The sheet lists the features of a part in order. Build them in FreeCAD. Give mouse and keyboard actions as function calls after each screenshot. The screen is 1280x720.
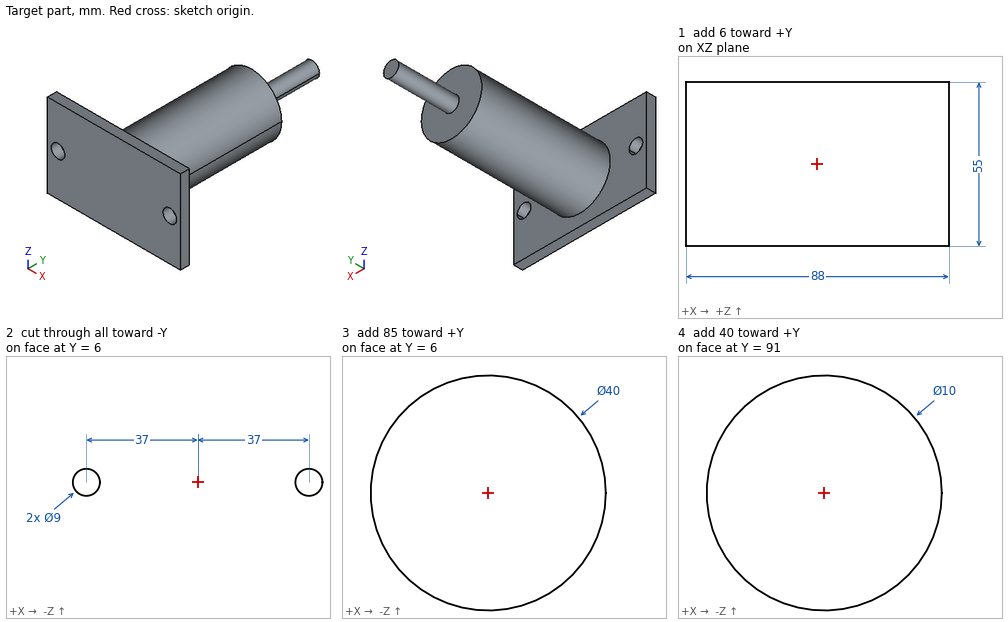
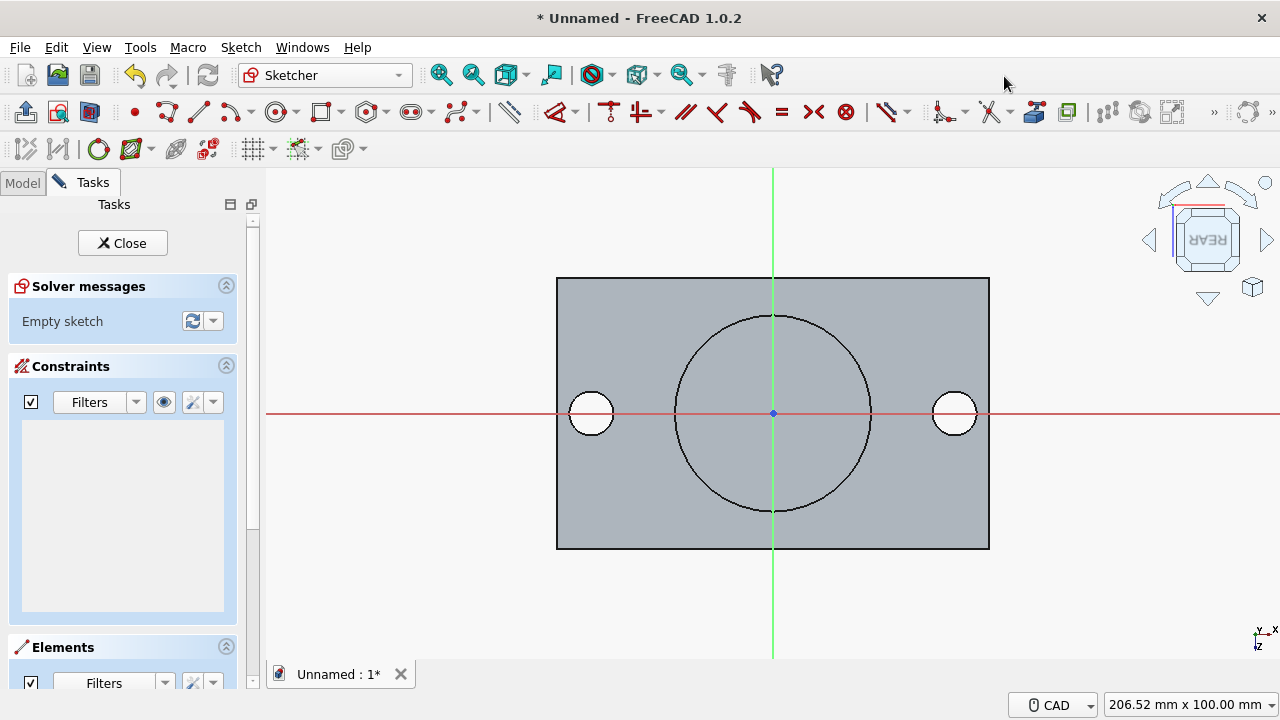
scroll(787, 413, up, 9)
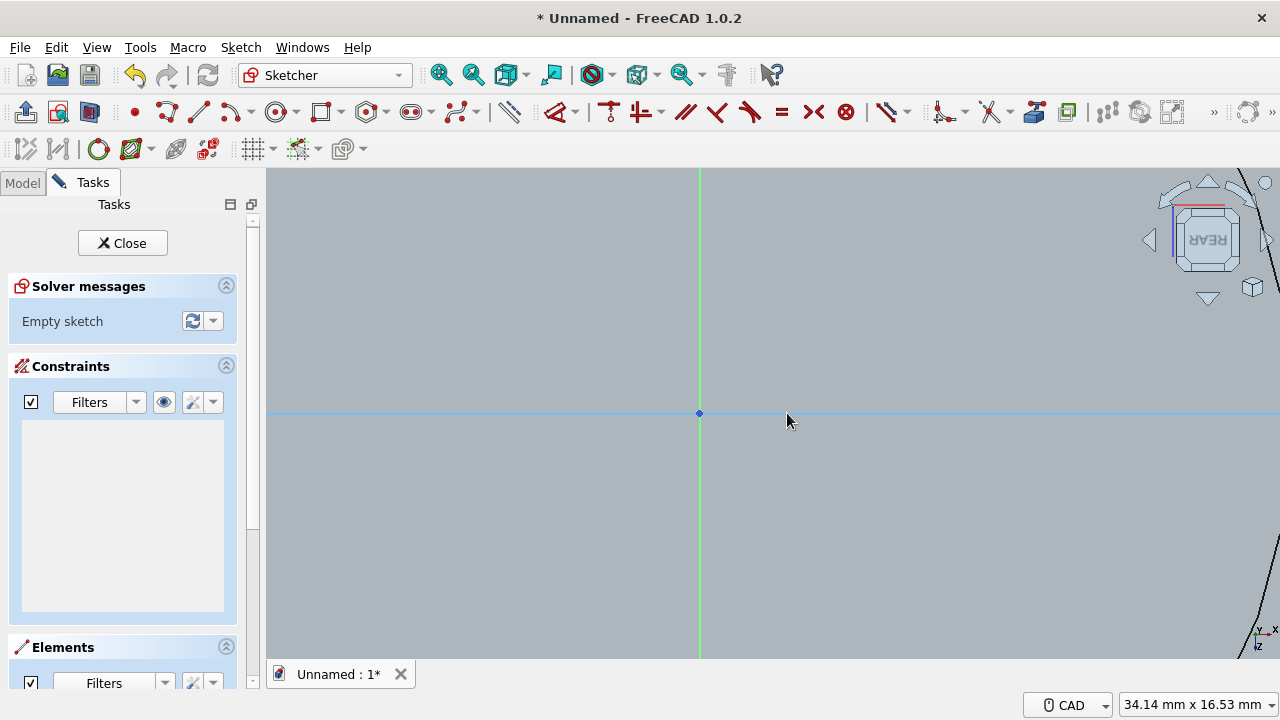
key(g)
key(c)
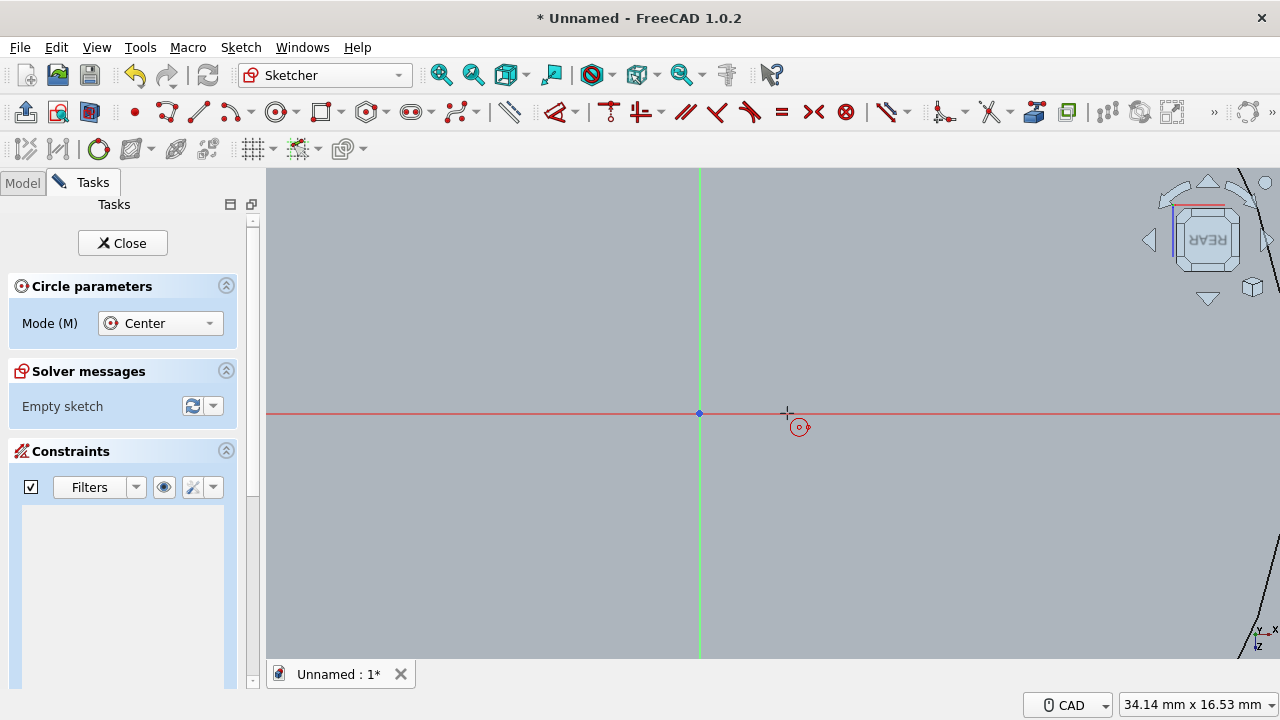
click(700, 413)
click(805, 308)
key(Escape)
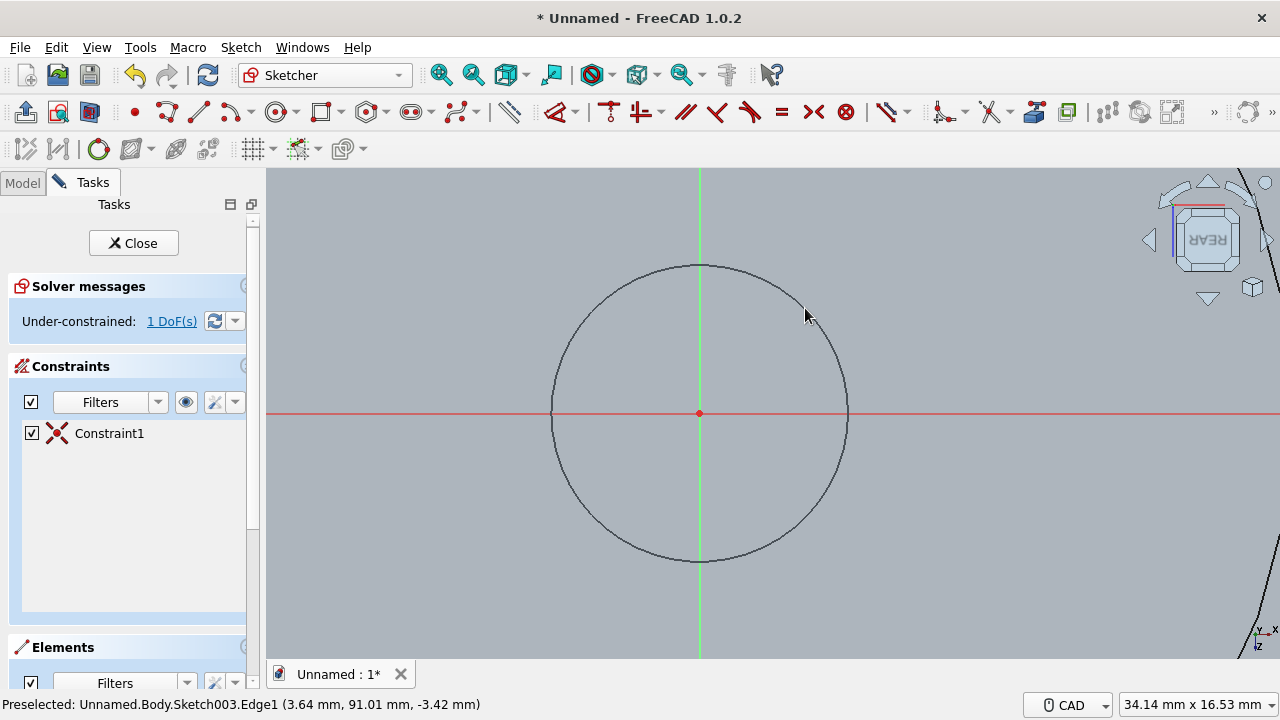
click(804, 308)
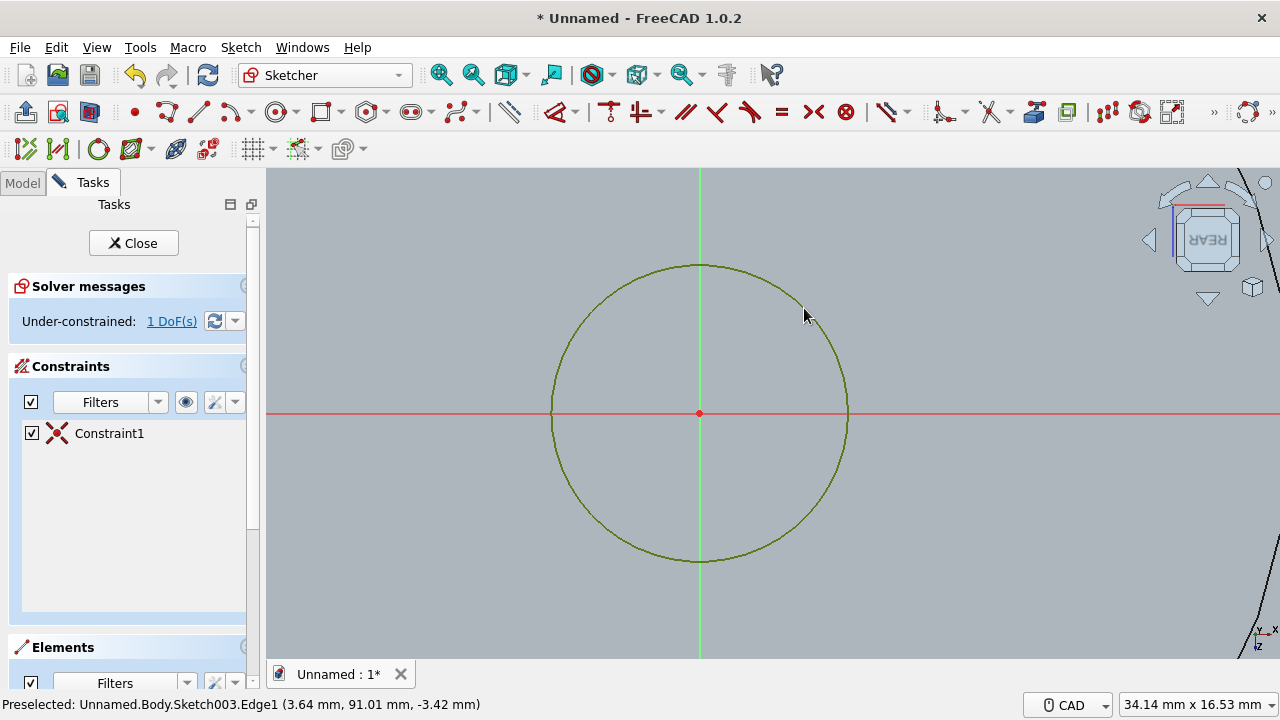
key(k)
key(o)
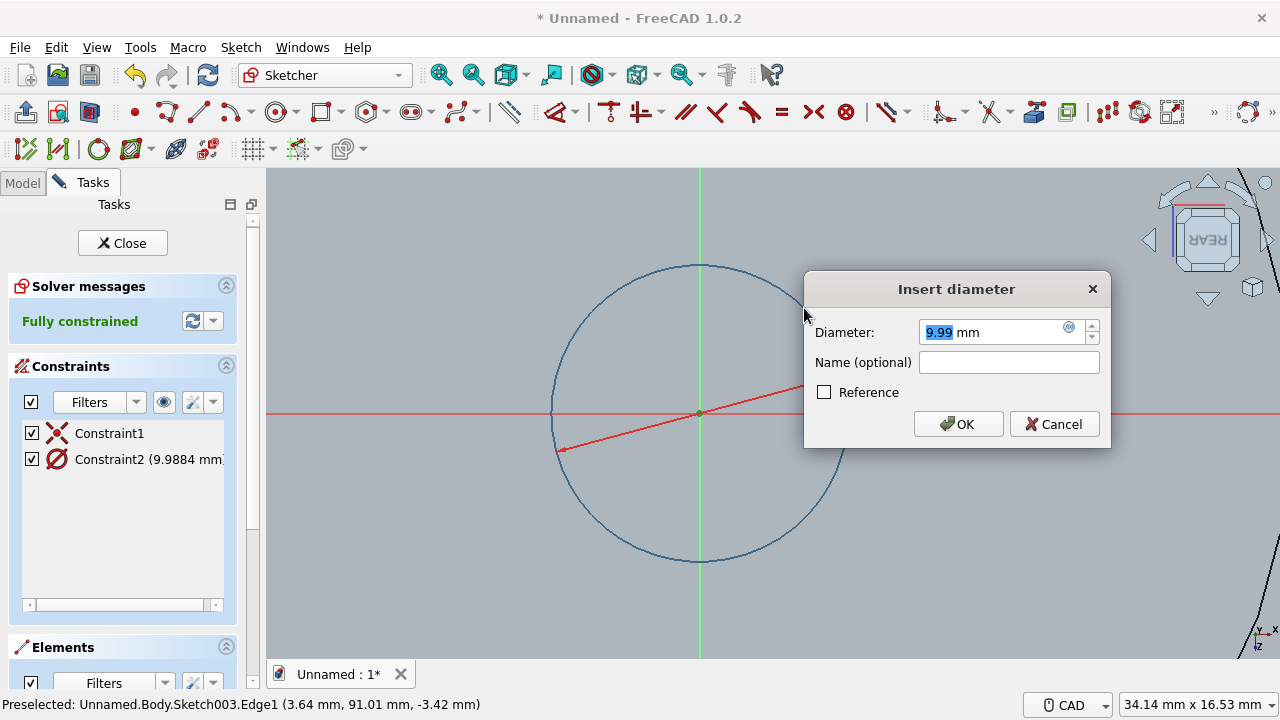
text(10)
key(Return)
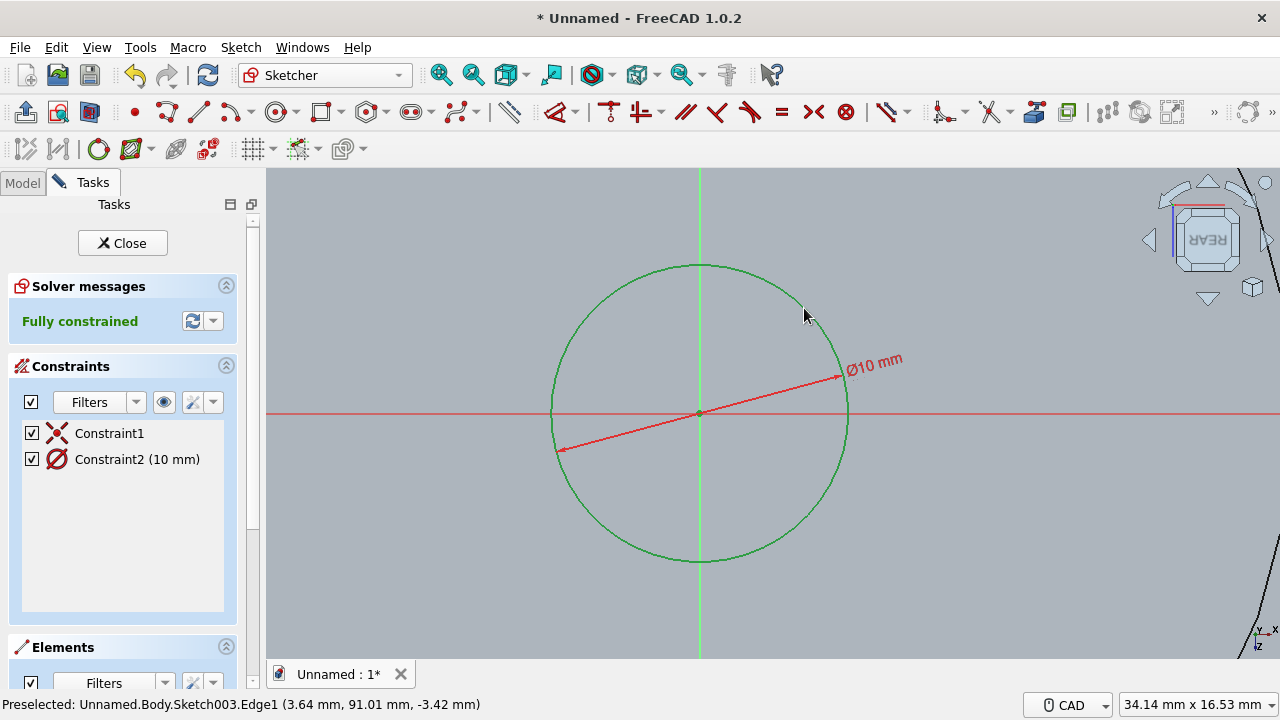
click(123, 243)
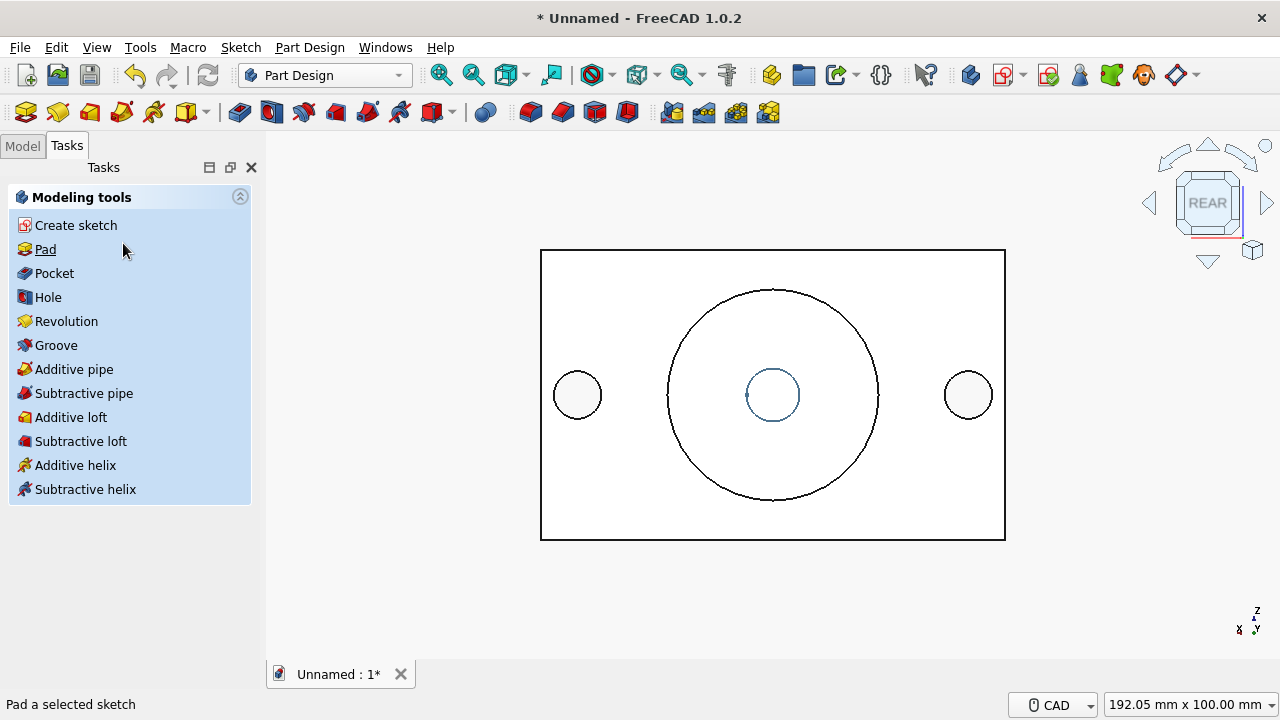
click(26, 112)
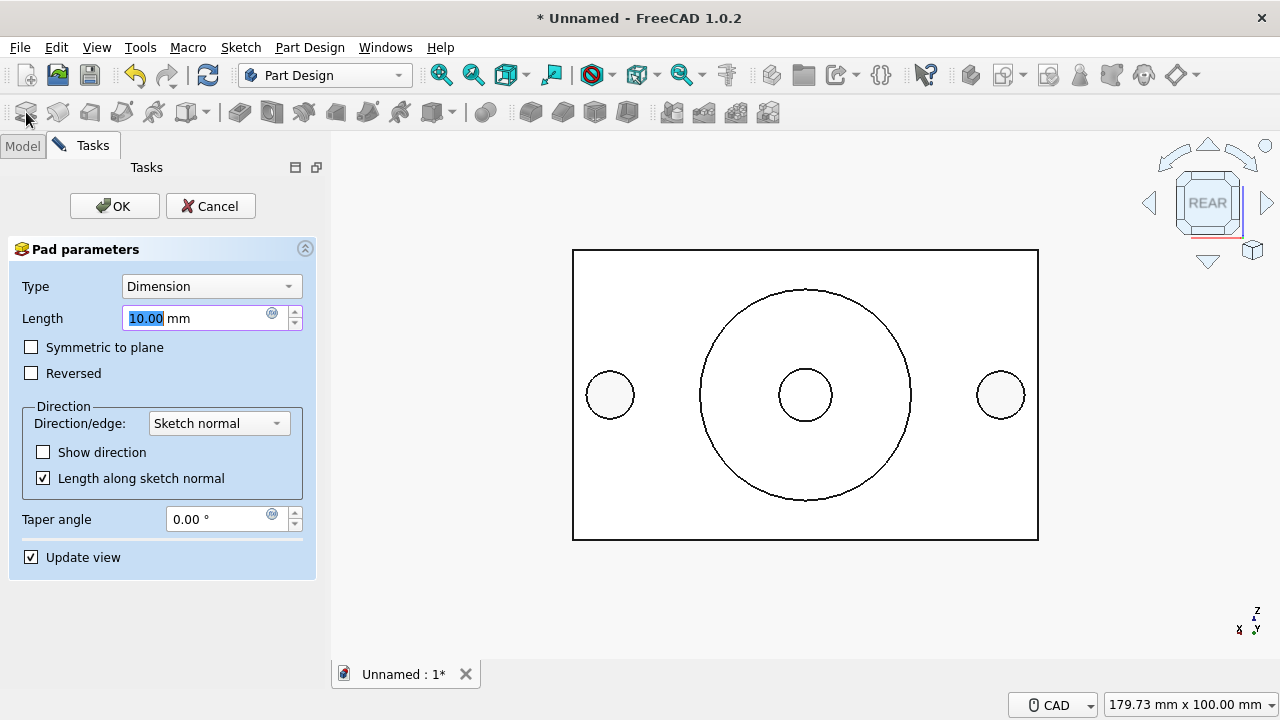
text(40)
key(Tab)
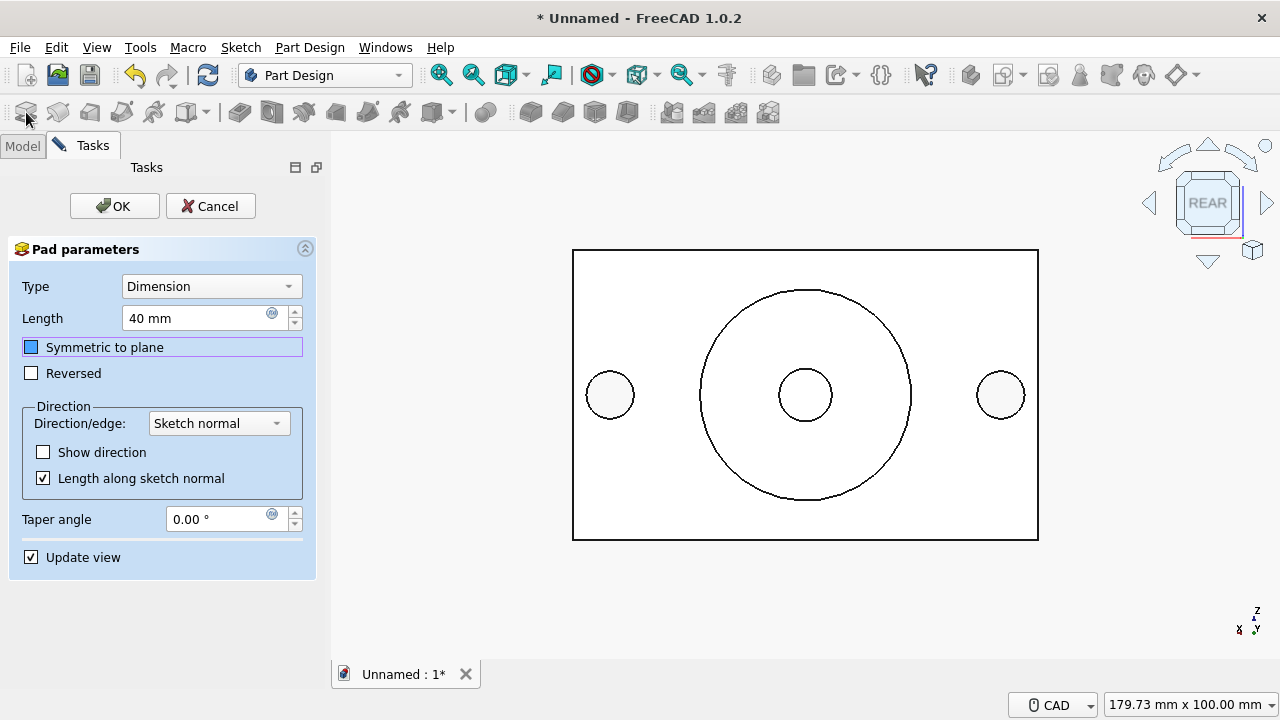
click(115, 206)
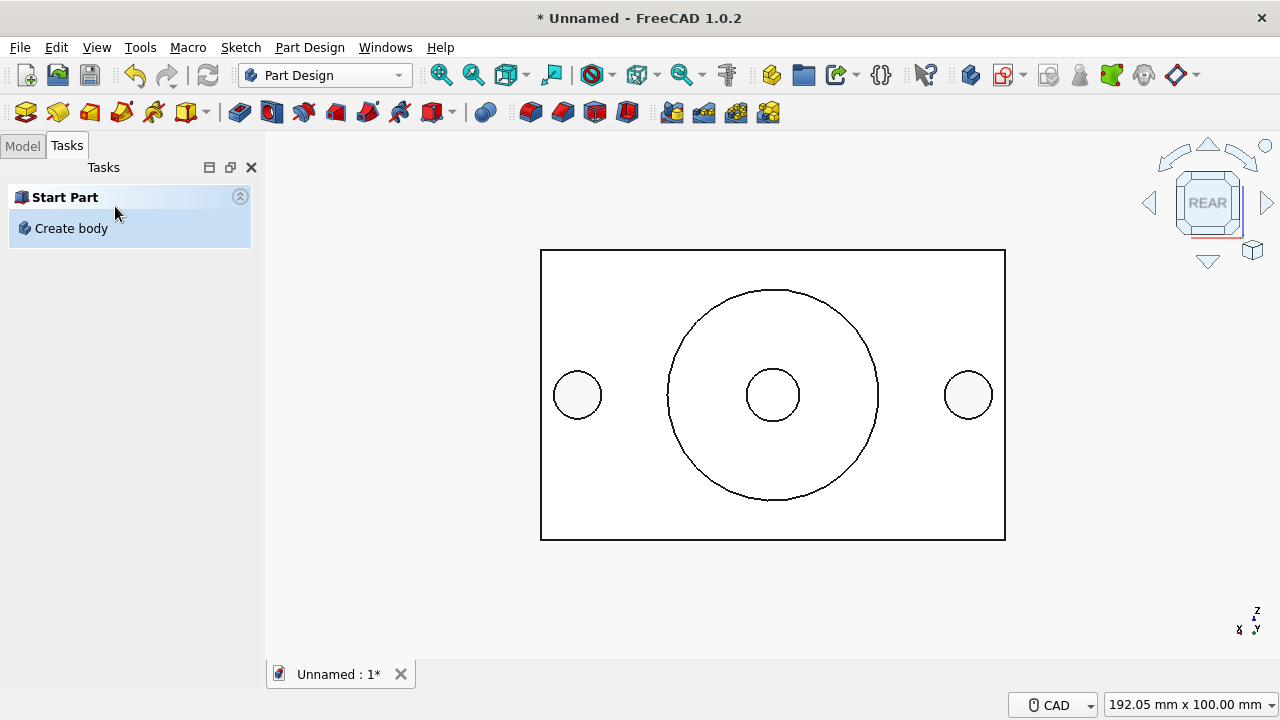
key(0)